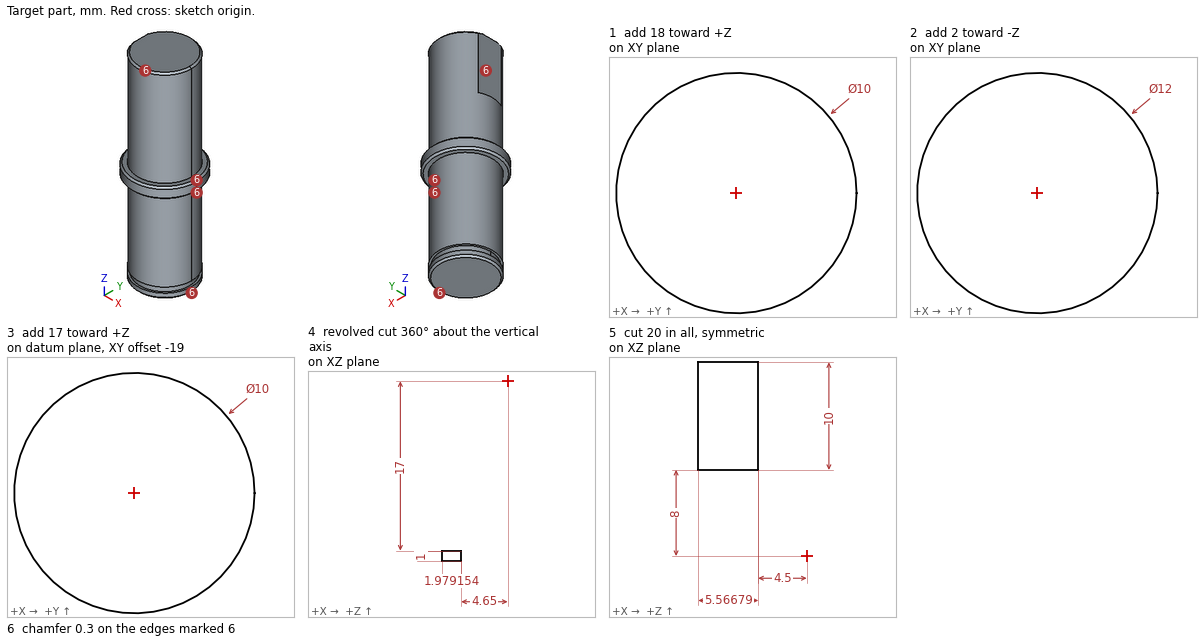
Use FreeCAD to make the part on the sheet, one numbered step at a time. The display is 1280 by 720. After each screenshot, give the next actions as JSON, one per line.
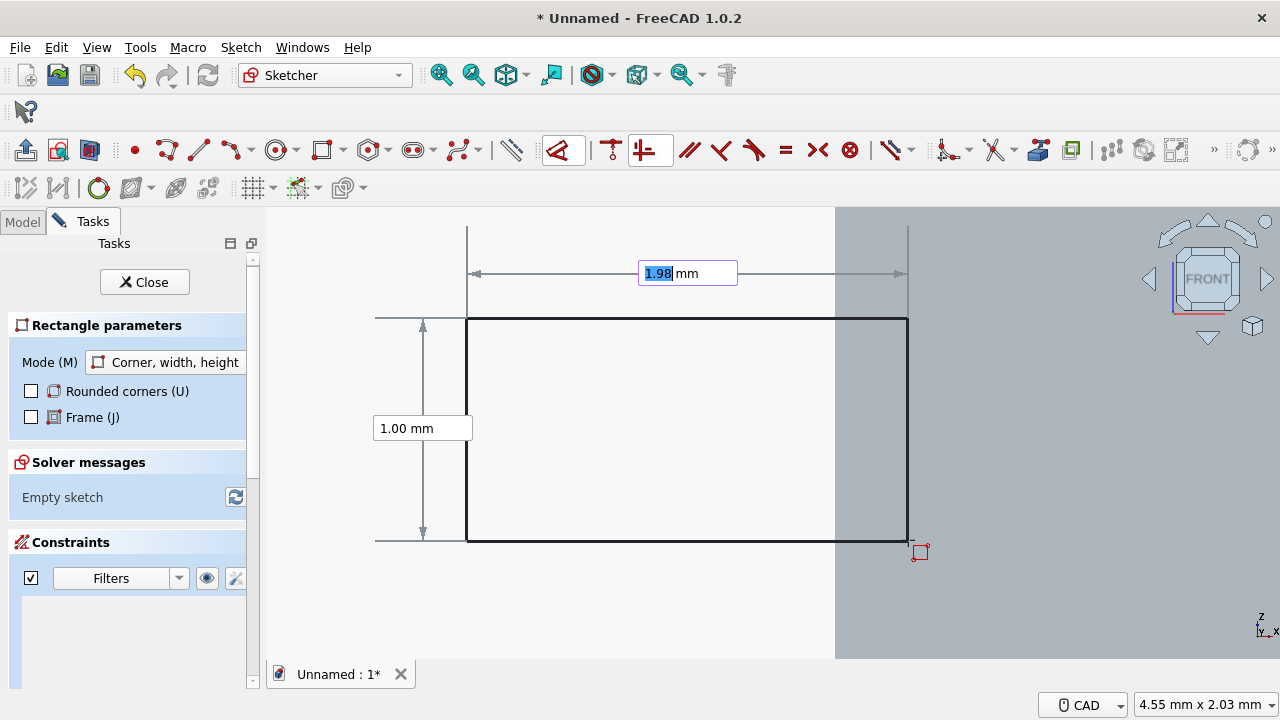
{"action": "type", "text": "1.979154"}
{"action": "key", "text": "Tab"}
{"action": "type", "text": "1"}
{"action": "key", "text": "Return"}
{"action": "key", "text": "Escape"}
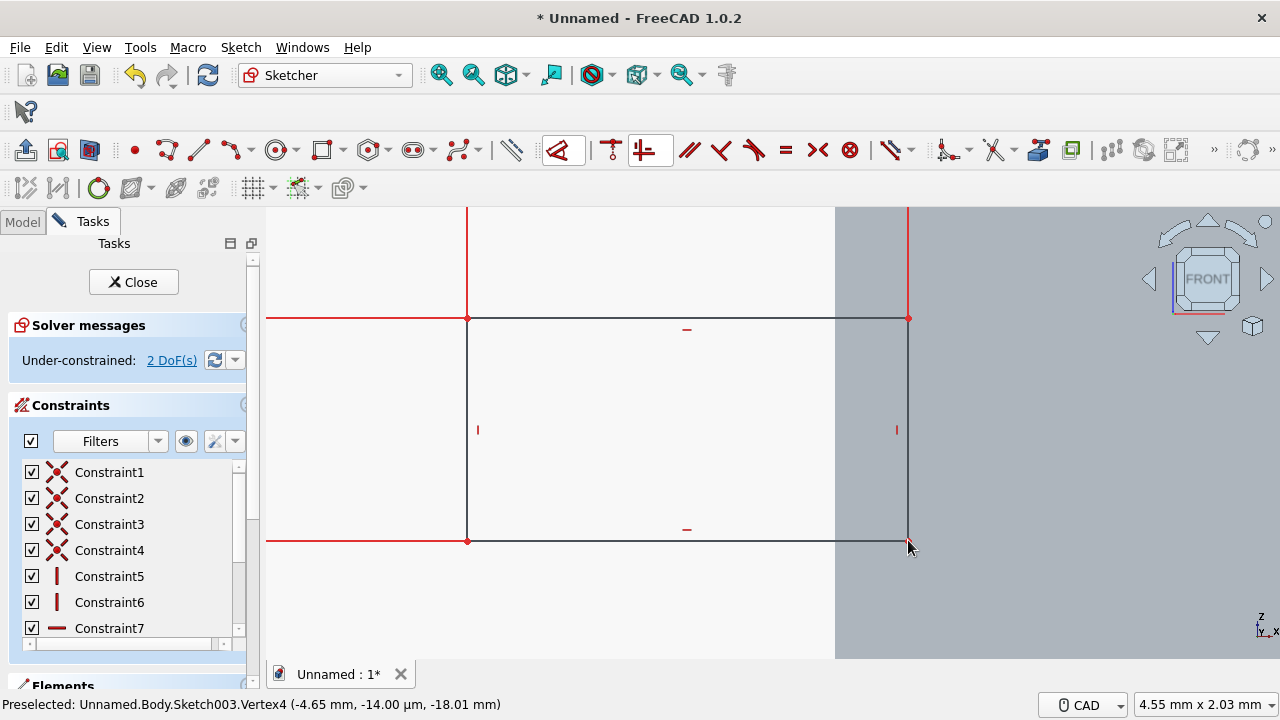
{"action": "left_click", "coordinate": [558, 150]}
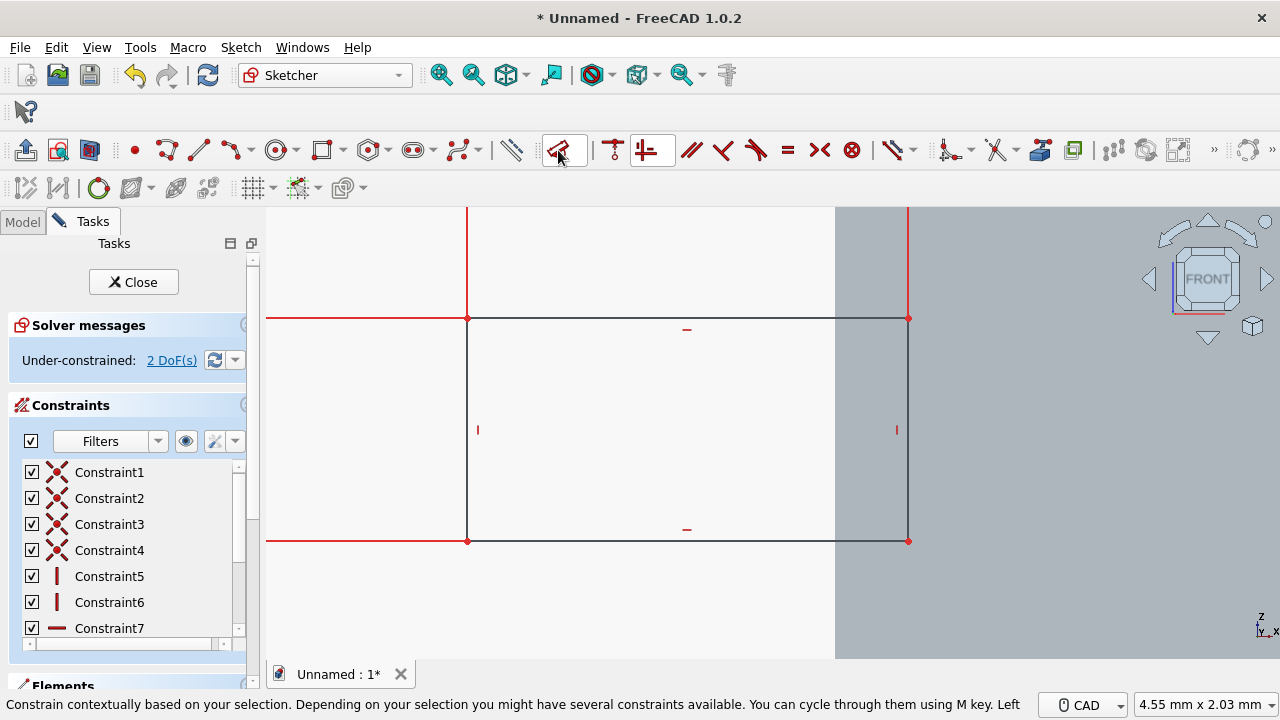
{"action": "left_click", "coordinate": [467, 318]}
{"action": "left_click", "coordinate": [433, 276]}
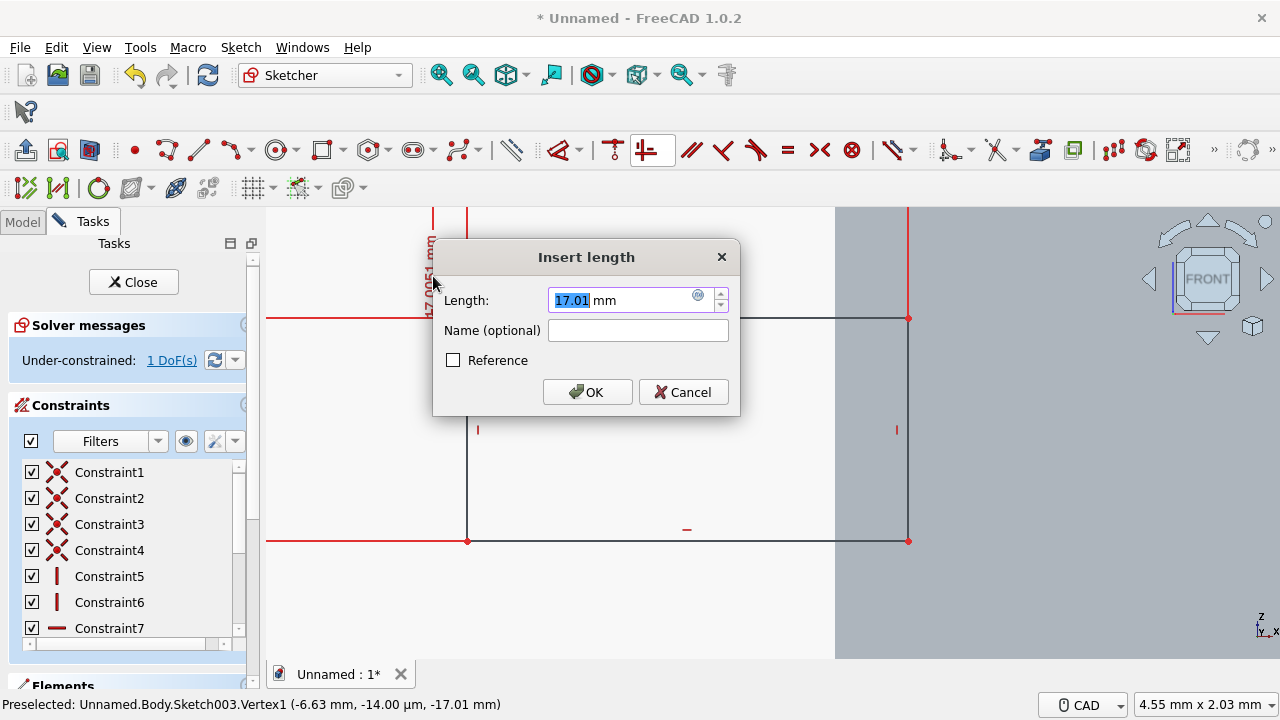
{"action": "type", "text": "17"}
{"action": "key", "text": "Return"}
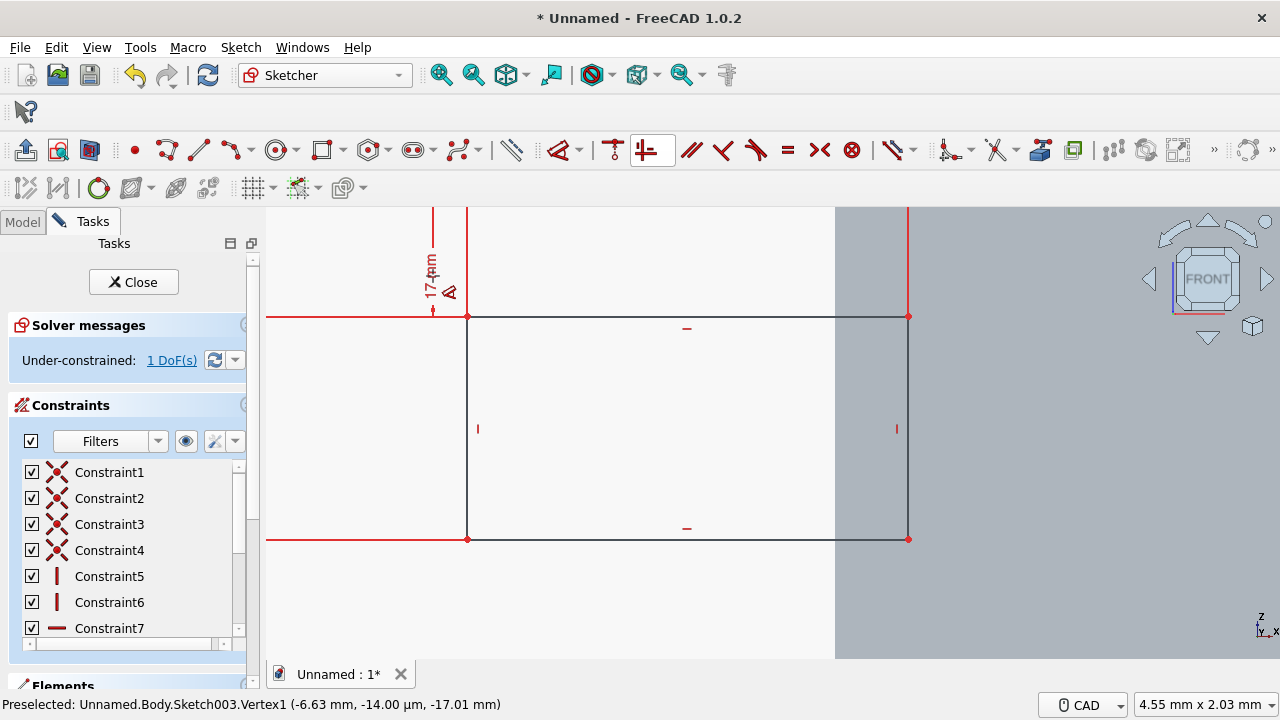
{"action": "left_click", "coordinate": [909, 540]}
{"action": "left_click", "coordinate": [1012, 574]}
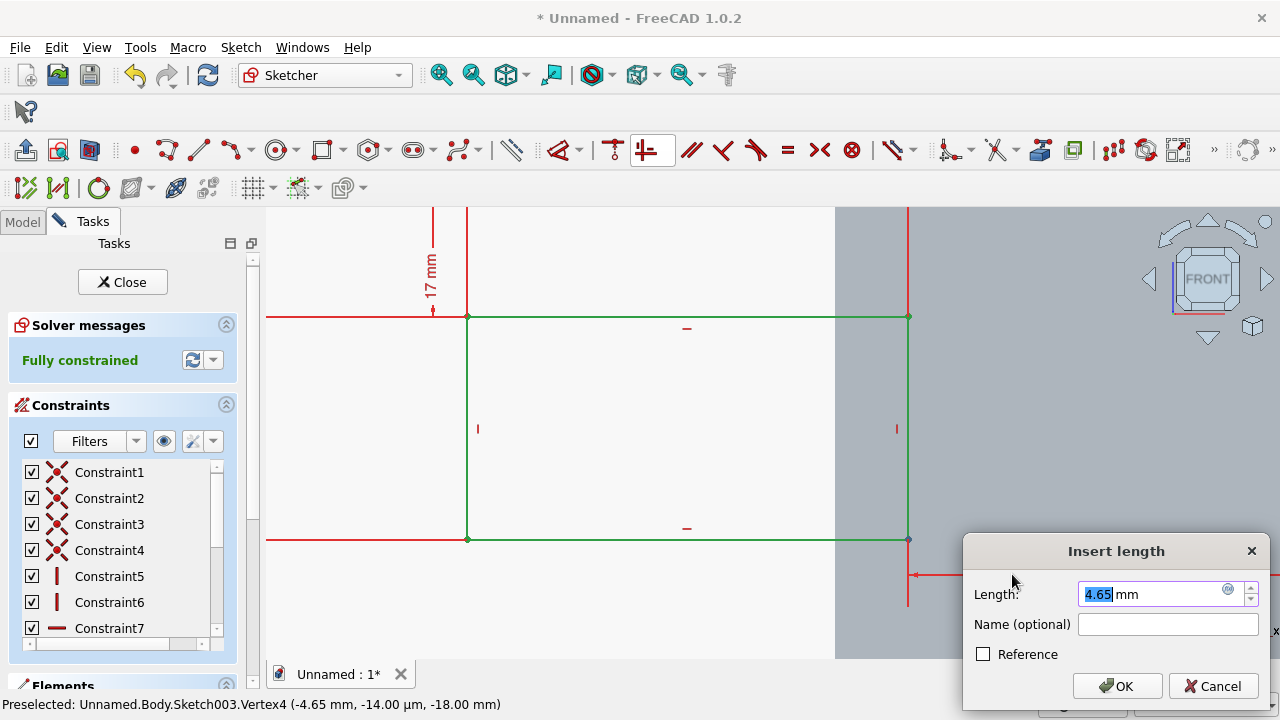
{"action": "type", "text": "4.65"}
{"action": "key", "text": "Return"}
{"action": "key", "text": "Escape"}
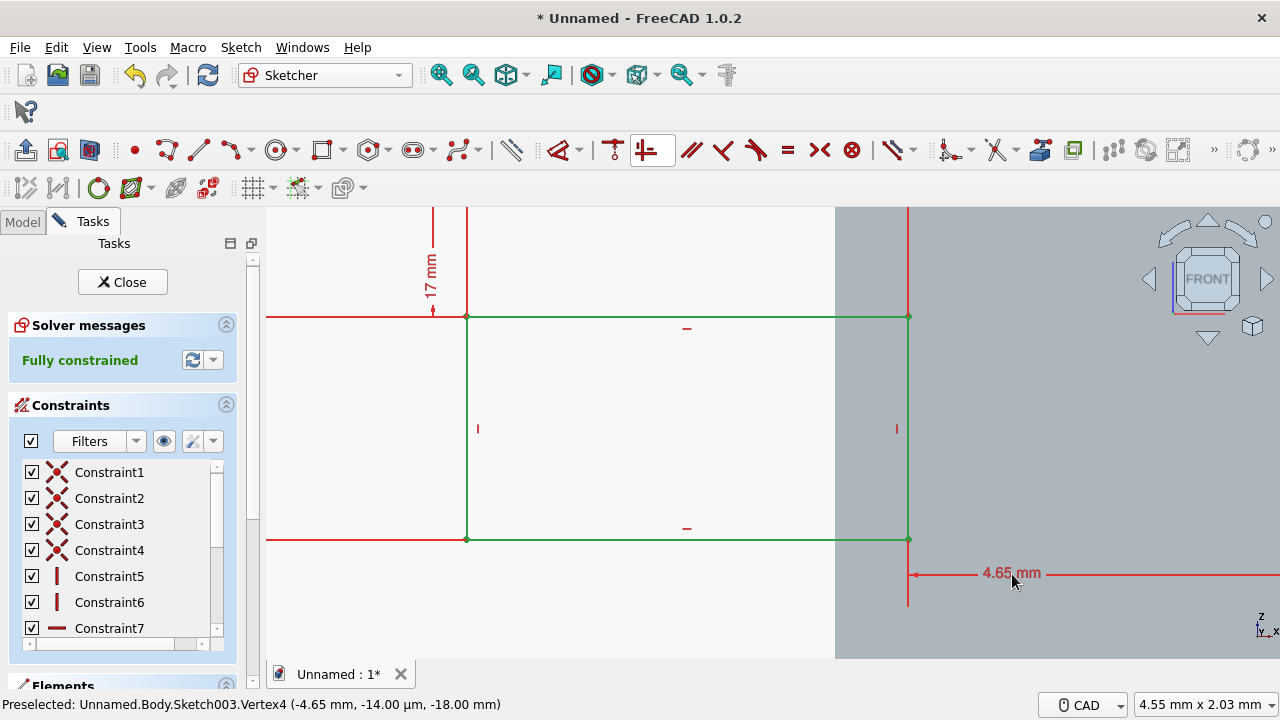
{"action": "left_click", "coordinate": [123, 282]}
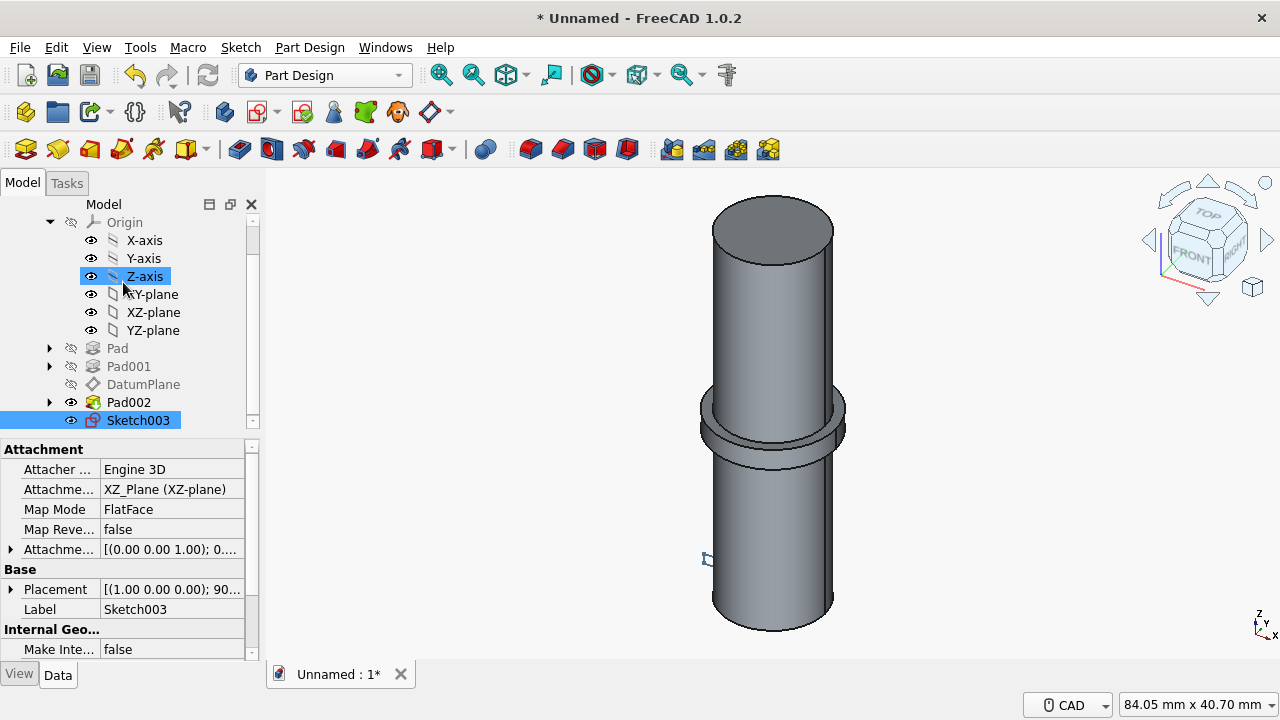
{"action": "left_click", "coordinate": [304, 150]}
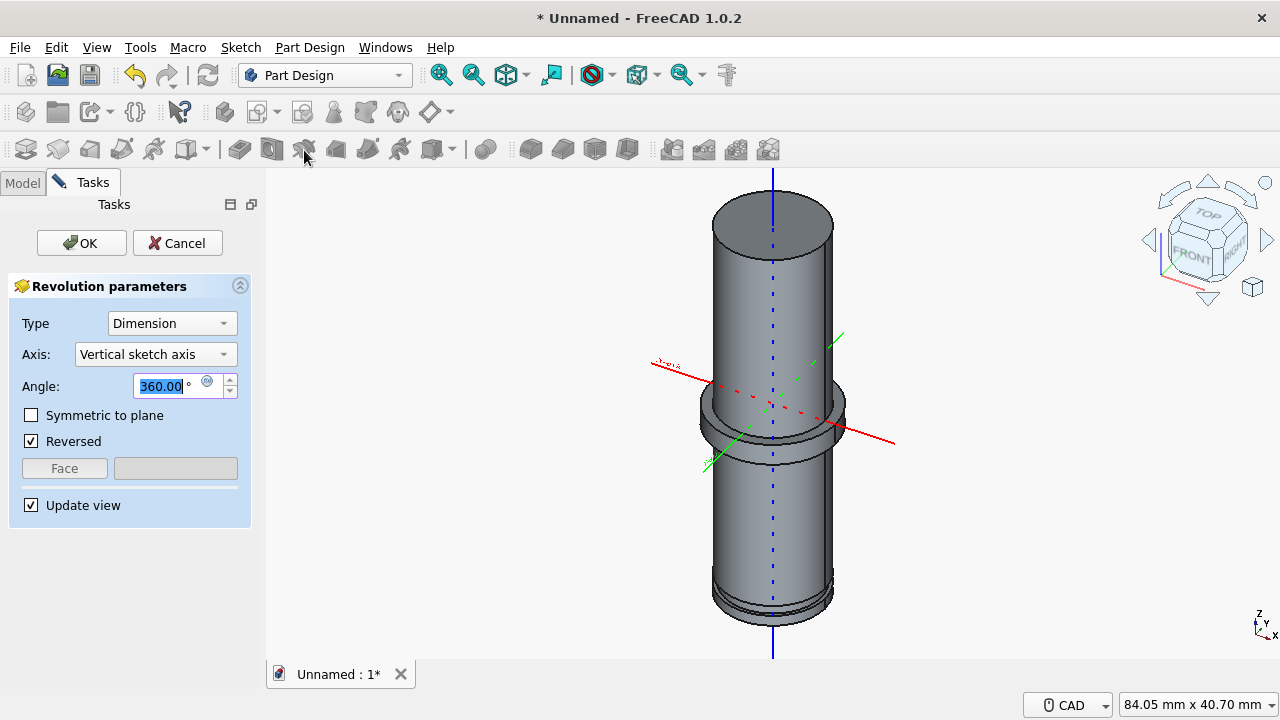
{"action": "left_click", "coordinate": [82, 243]}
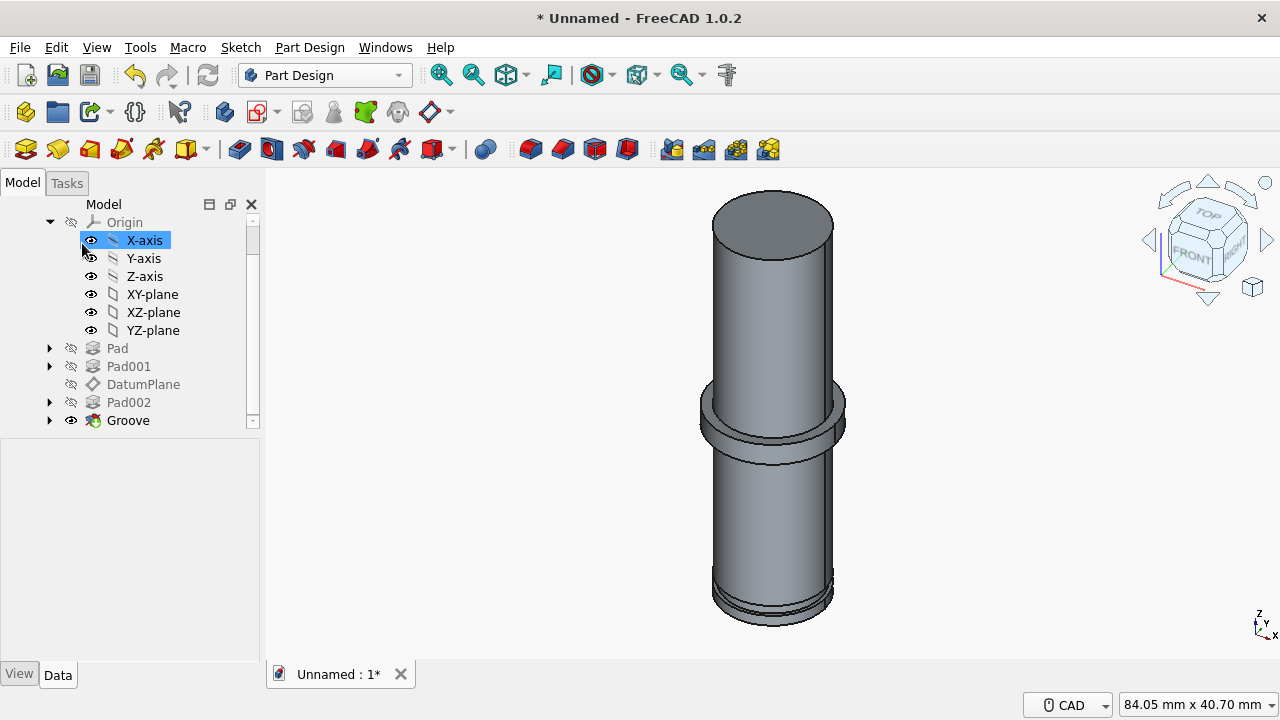
{"action": "left_click", "coordinate": [258, 112]}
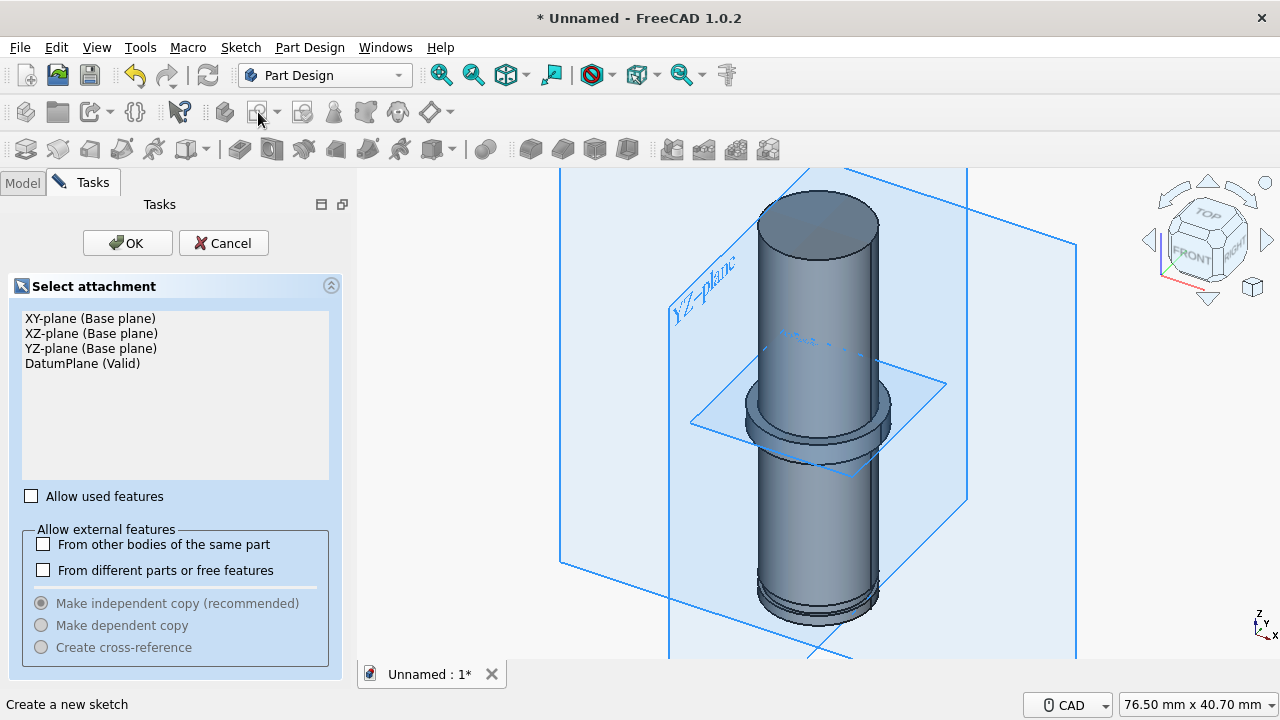
{"action": "left_click", "coordinate": [82, 334]}